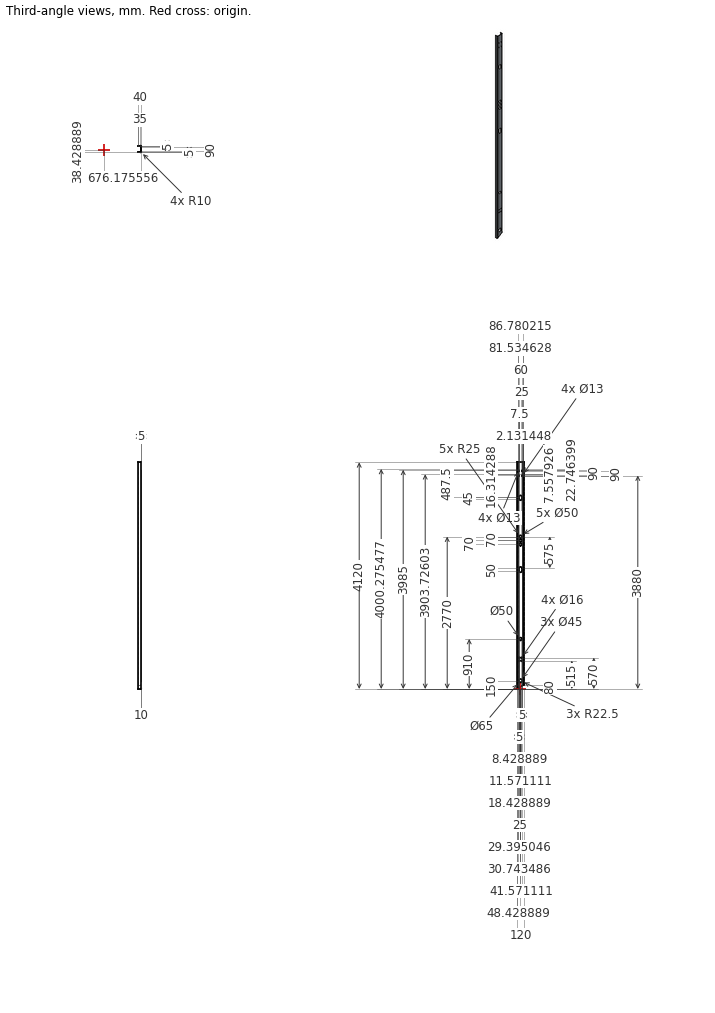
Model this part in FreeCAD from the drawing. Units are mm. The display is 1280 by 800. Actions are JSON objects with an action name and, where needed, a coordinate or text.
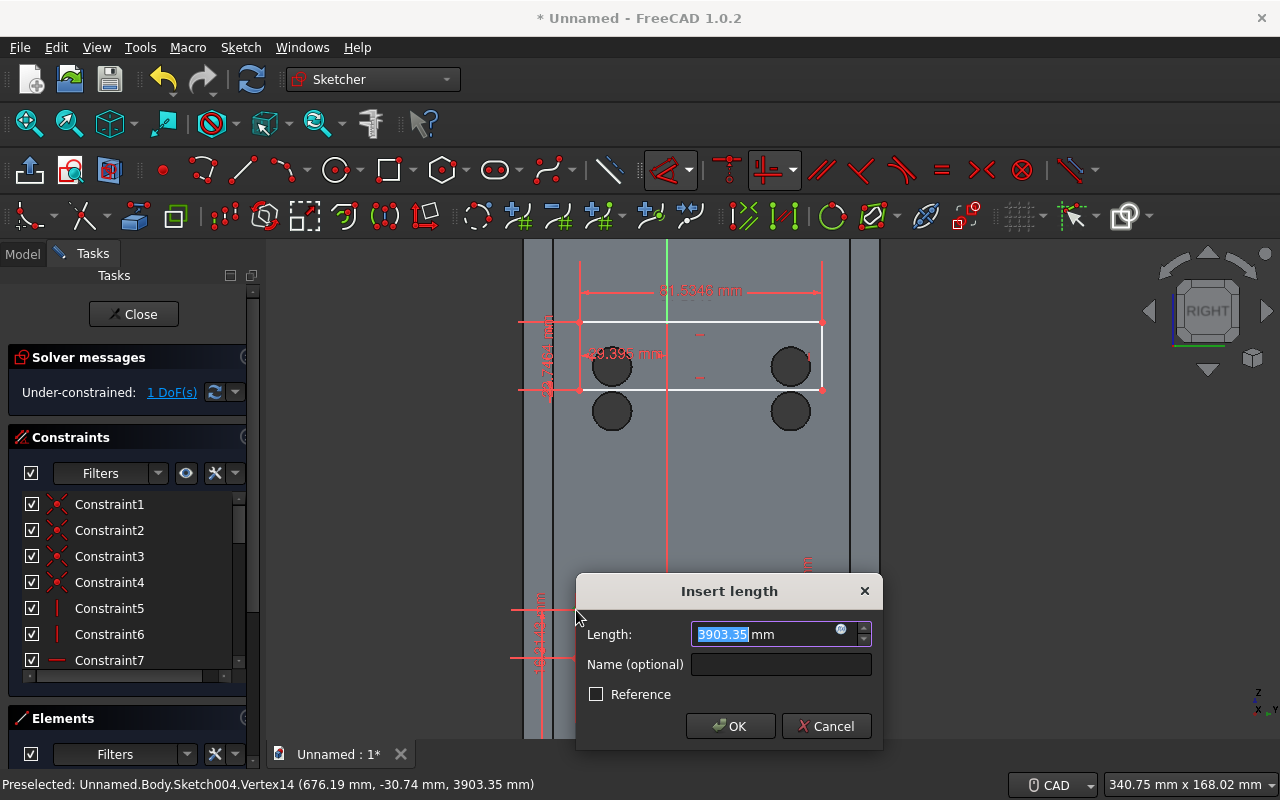
{"action": "type", "text": "3903.72603"}
{"action": "key", "text": "Return"}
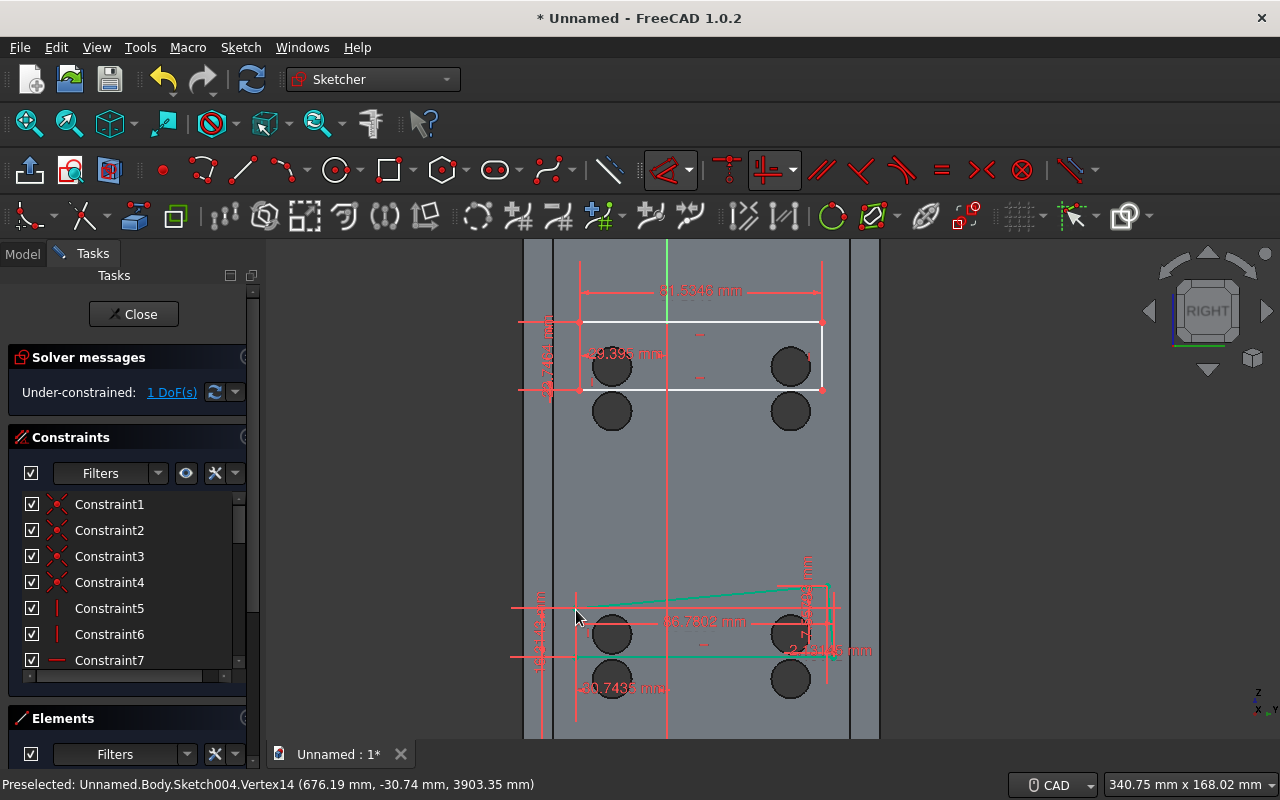
{"action": "left_click", "coordinate": [580, 322]}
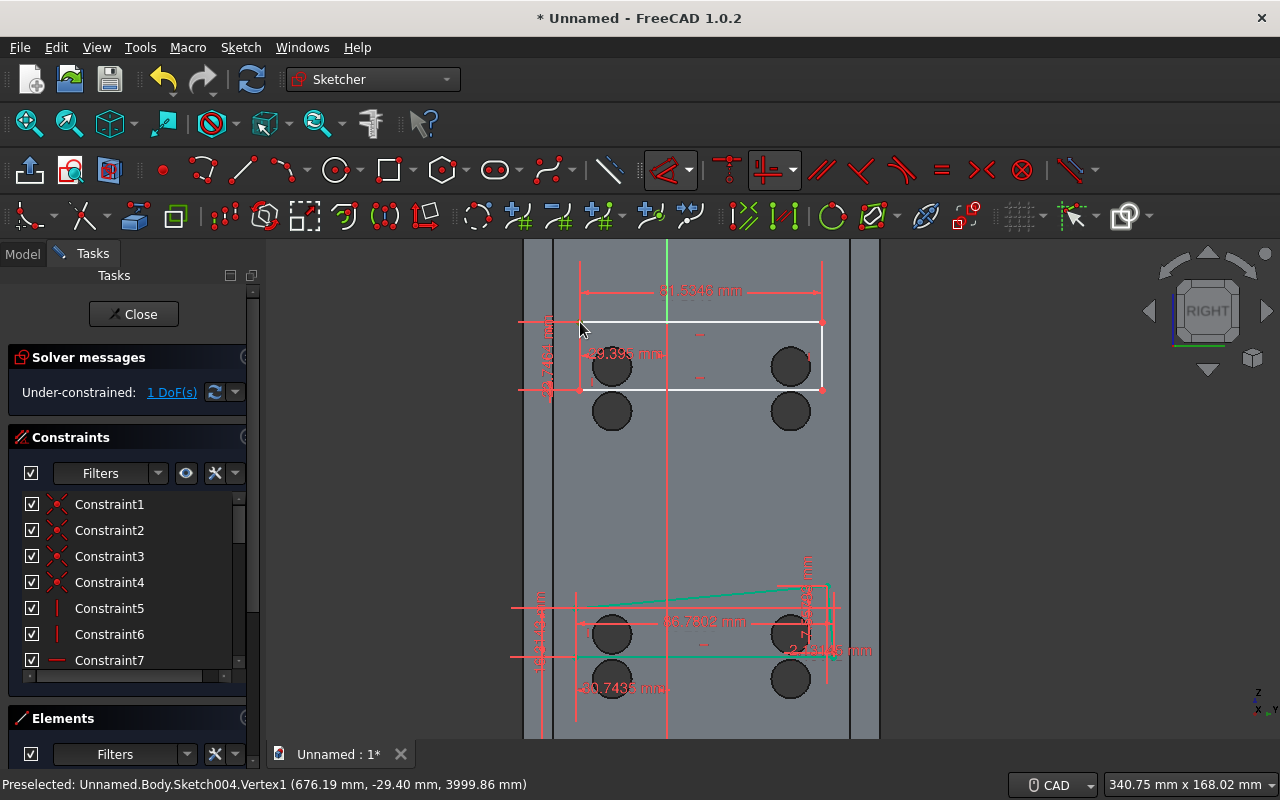
{"action": "left_click", "coordinate": [692, 170]}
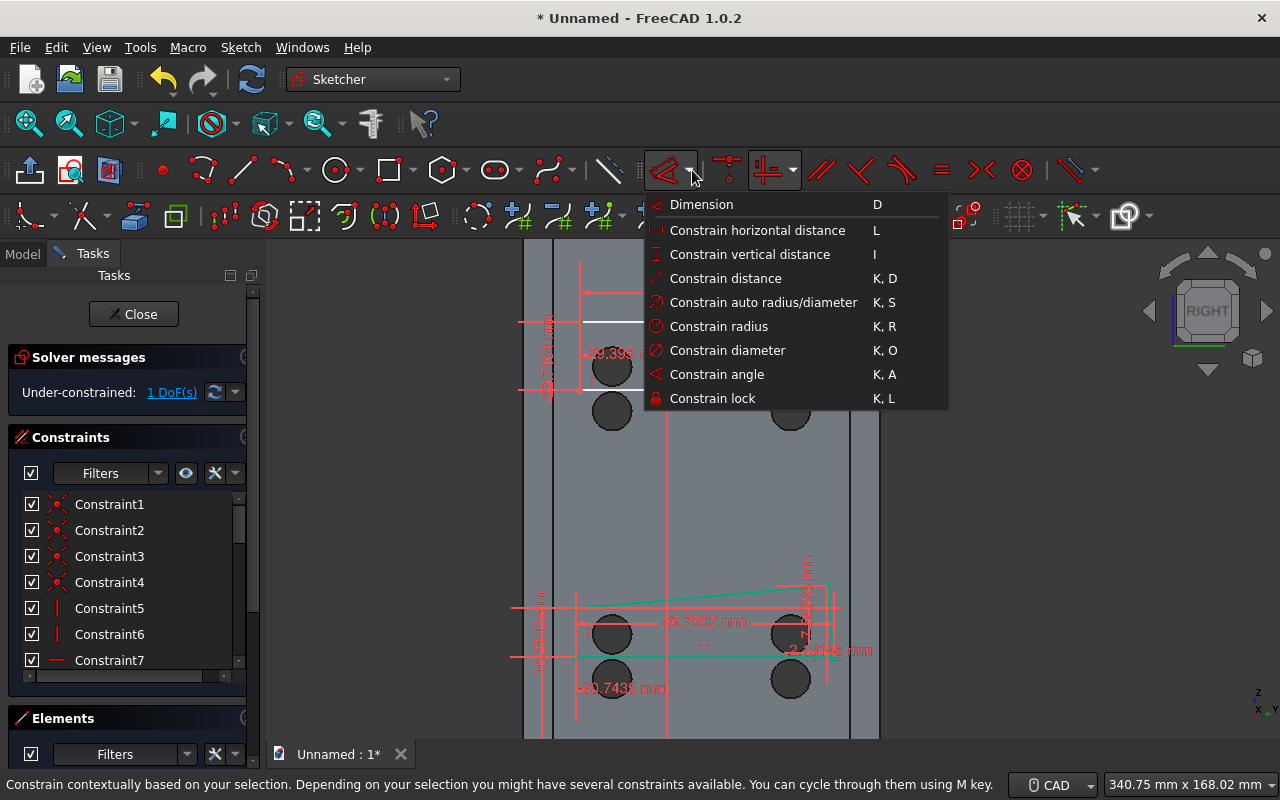
{"action": "left_click", "coordinate": [797, 254]}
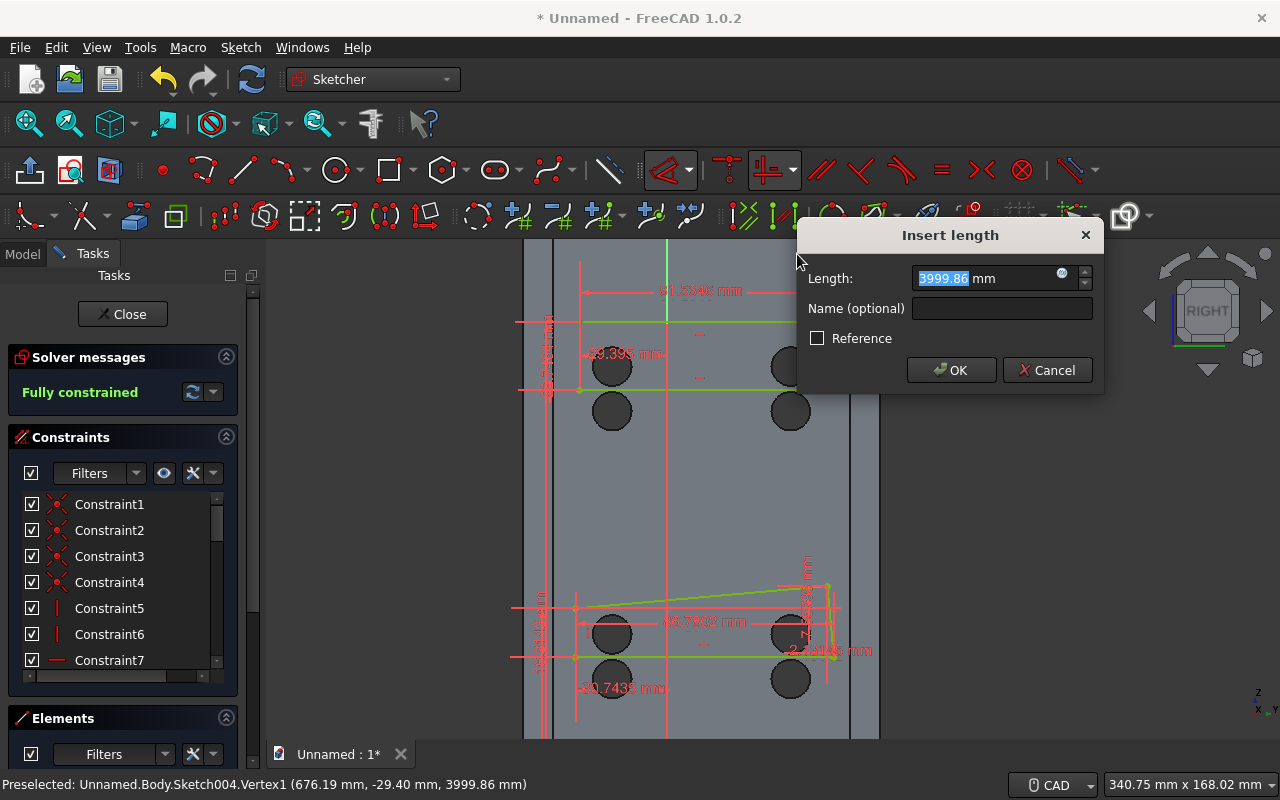
{"action": "type", "text": "4000.275477"}
{"action": "key", "text": "Return"}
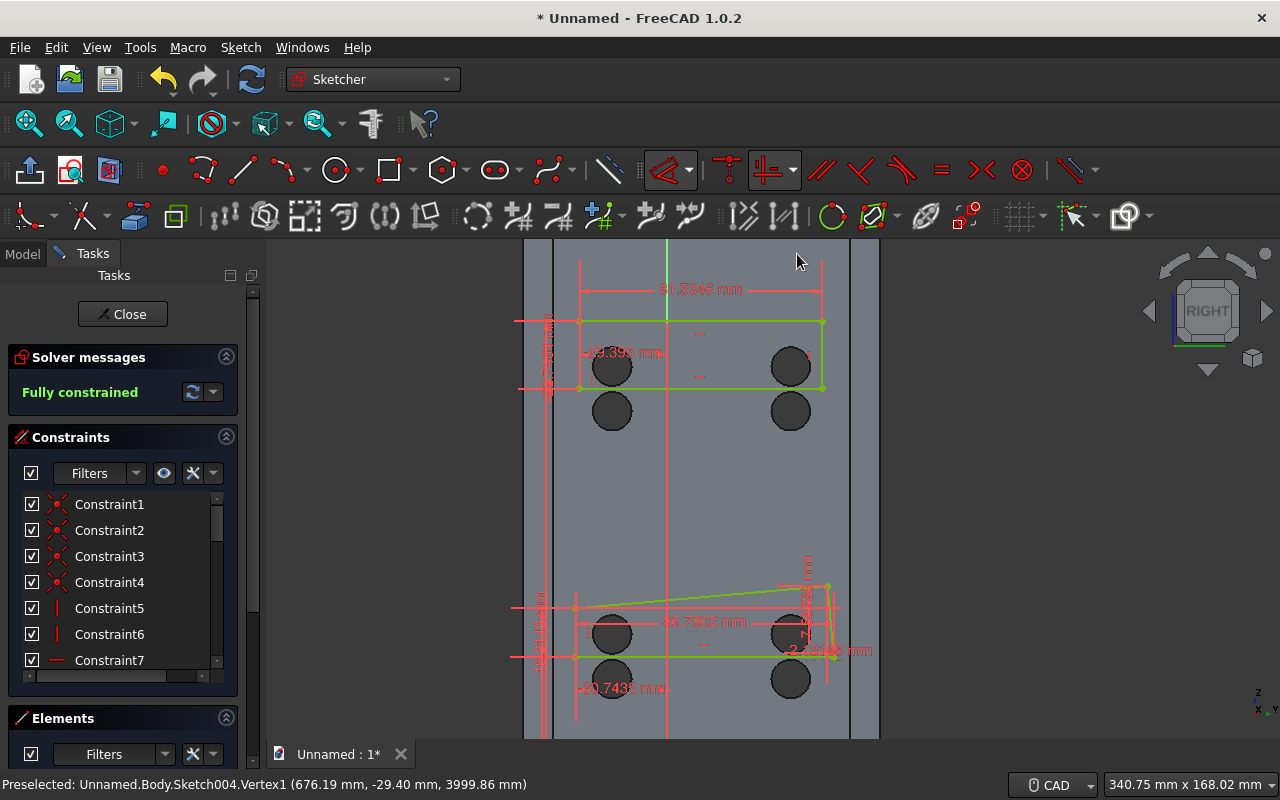
{"action": "left_click", "coordinate": [123, 314]}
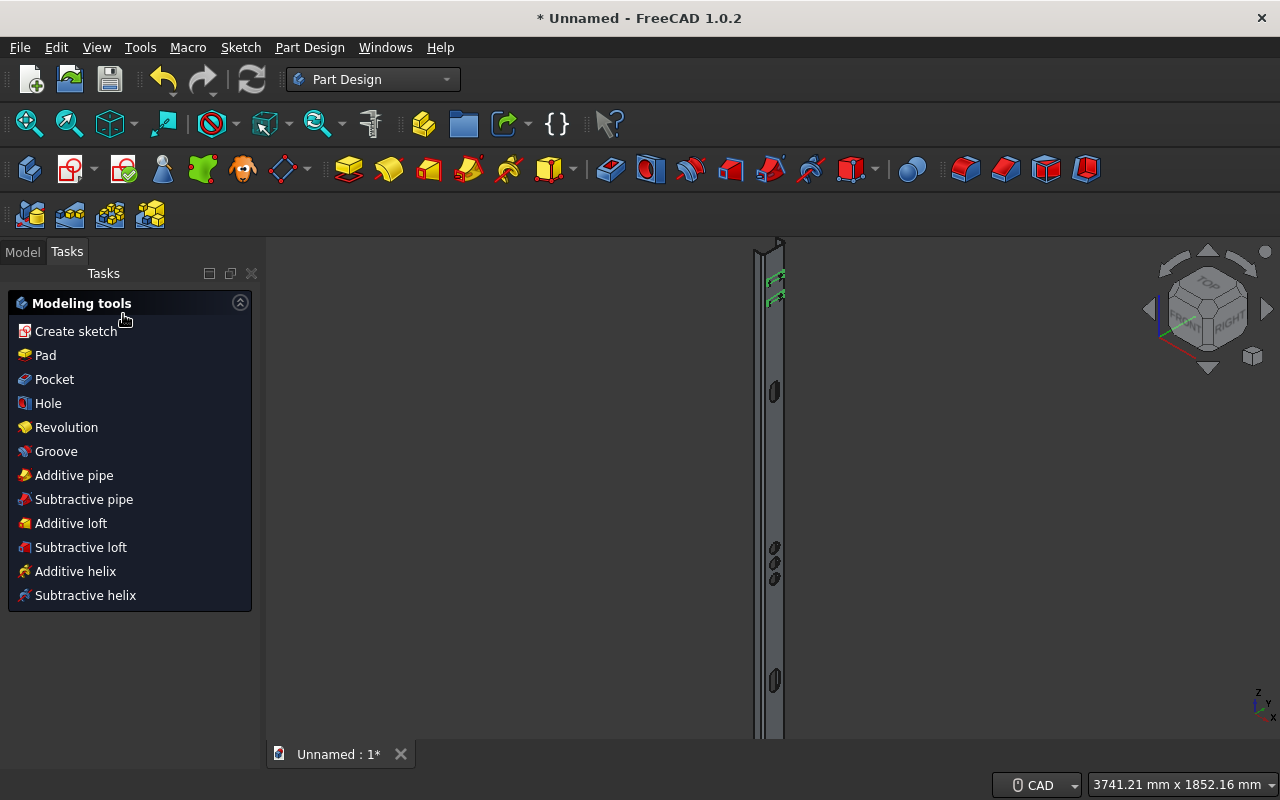
{"action": "left_click", "coordinate": [350, 170]}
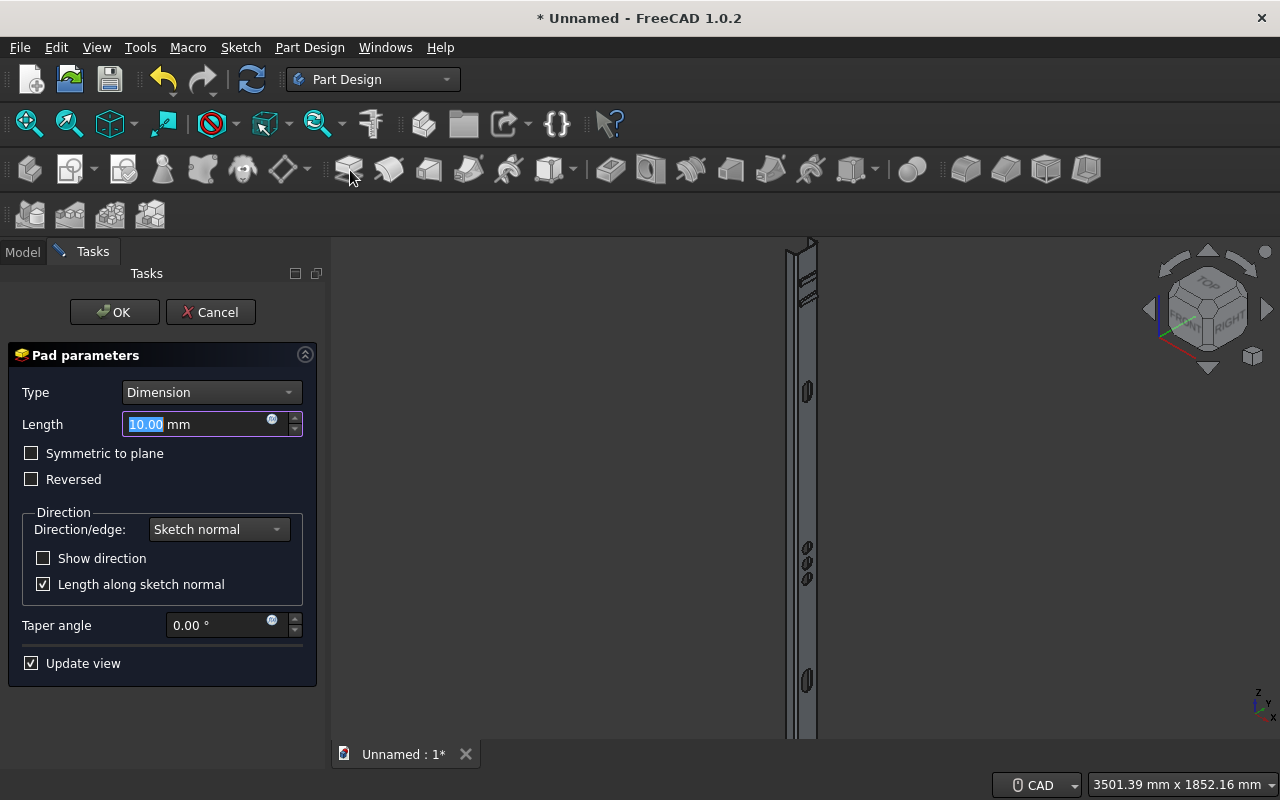
{"action": "type", "text": "5"}
{"action": "key", "text": "Tab"}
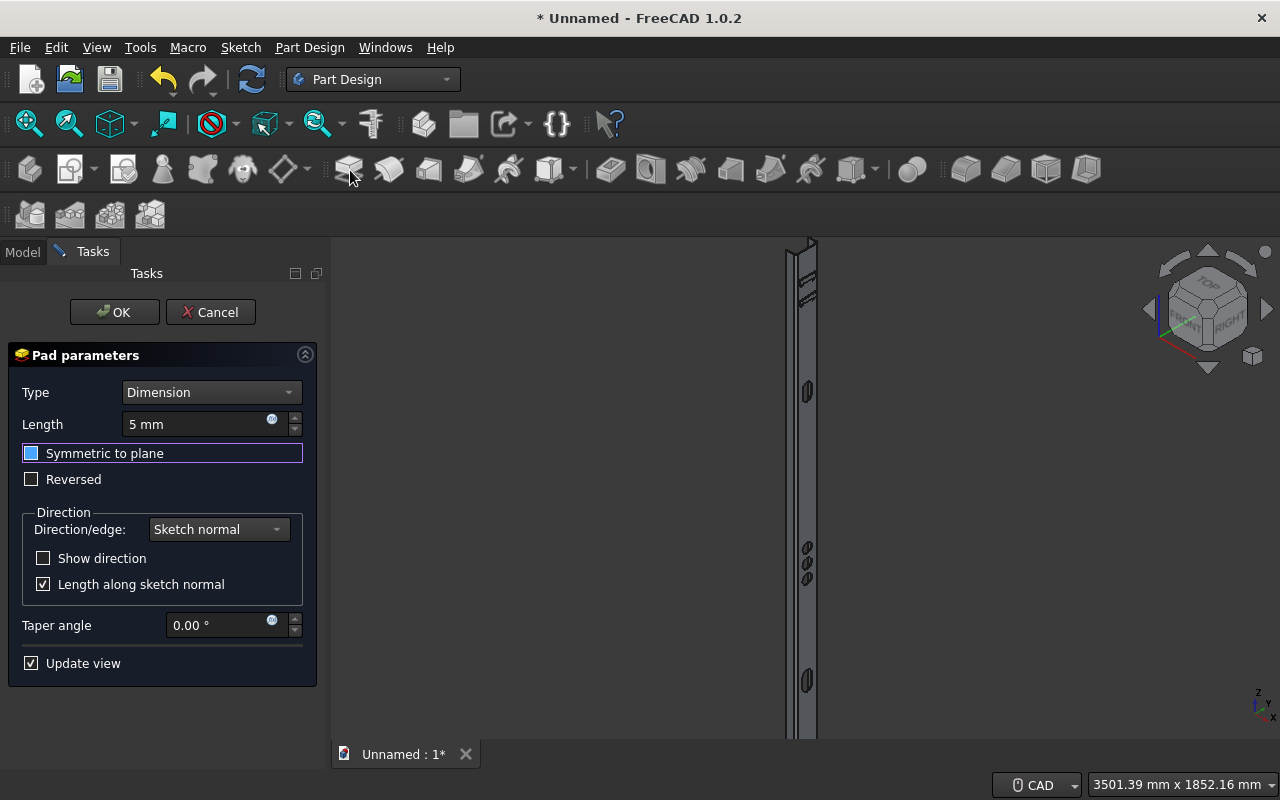
{"action": "left_click", "coordinate": [30, 479]}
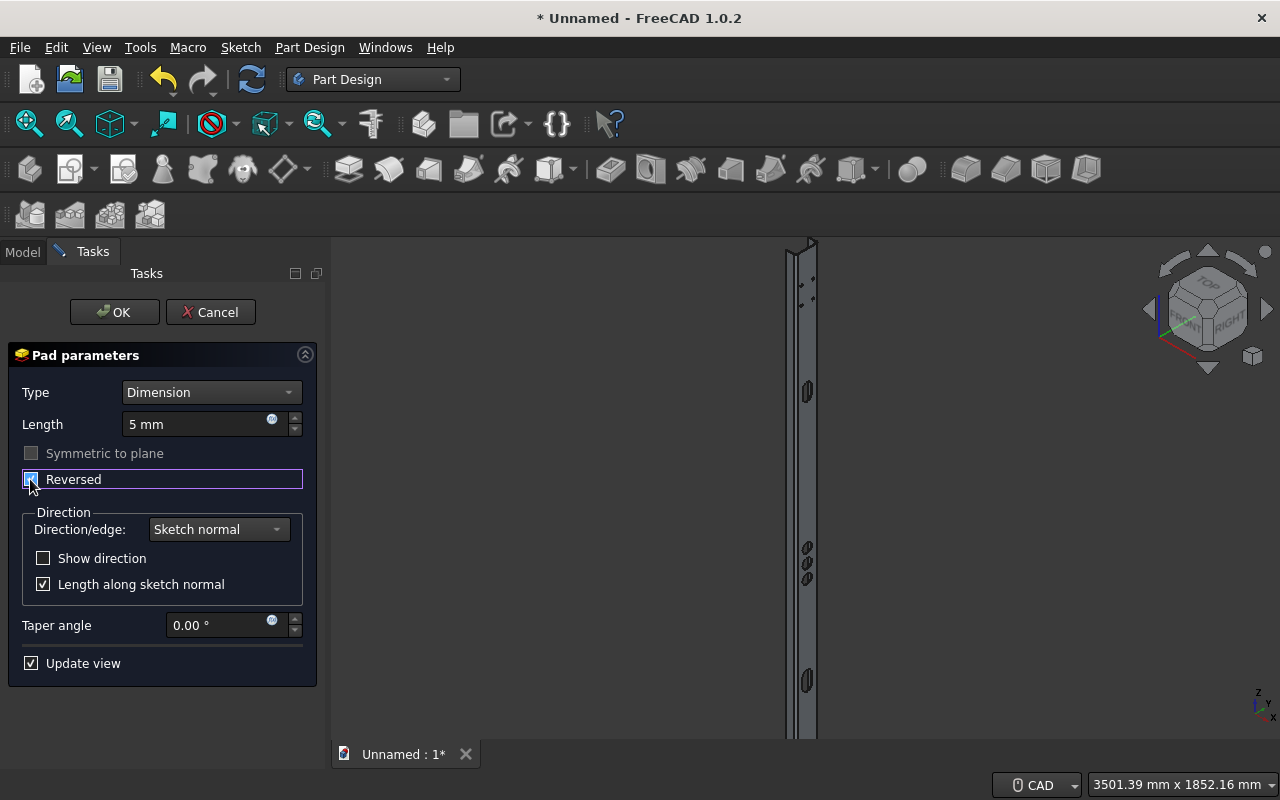
{"action": "left_click", "coordinate": [115, 312]}